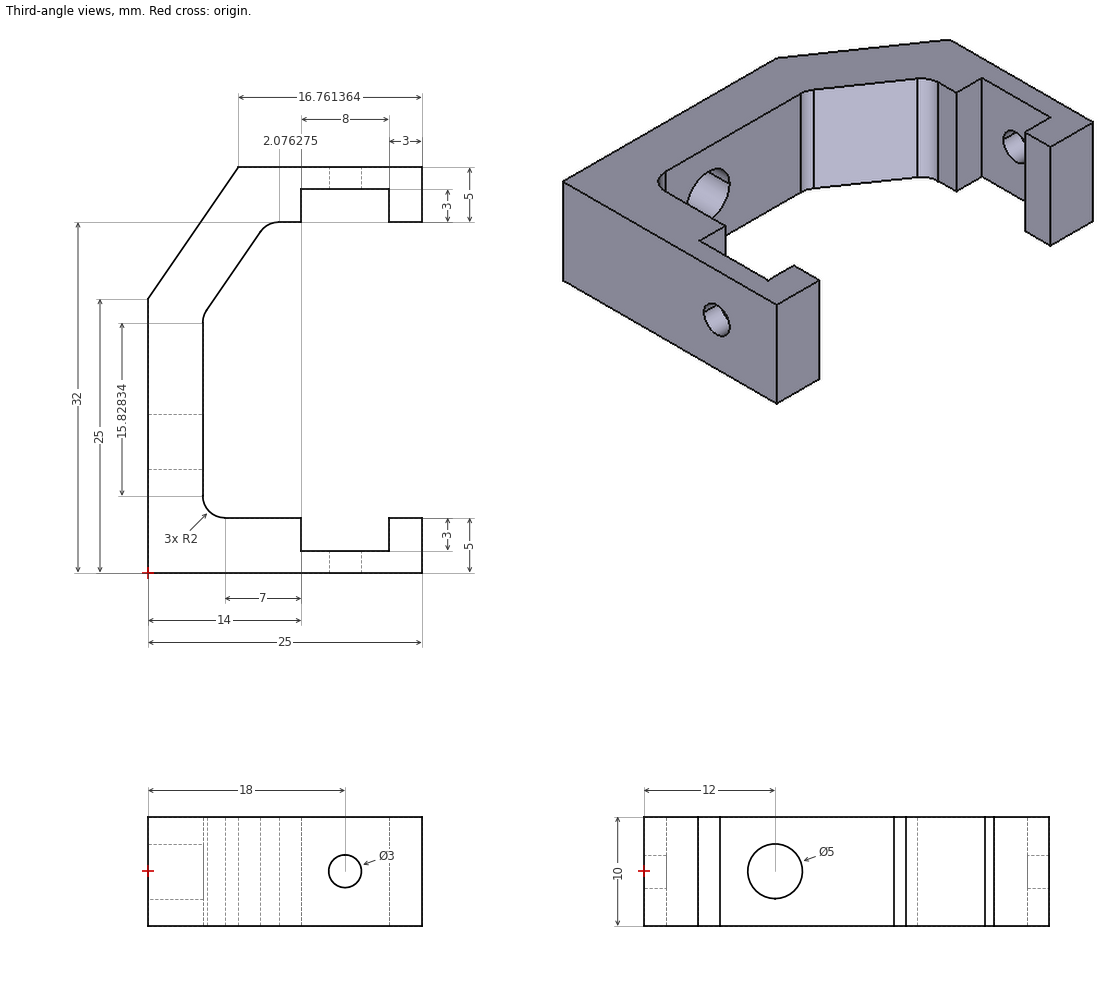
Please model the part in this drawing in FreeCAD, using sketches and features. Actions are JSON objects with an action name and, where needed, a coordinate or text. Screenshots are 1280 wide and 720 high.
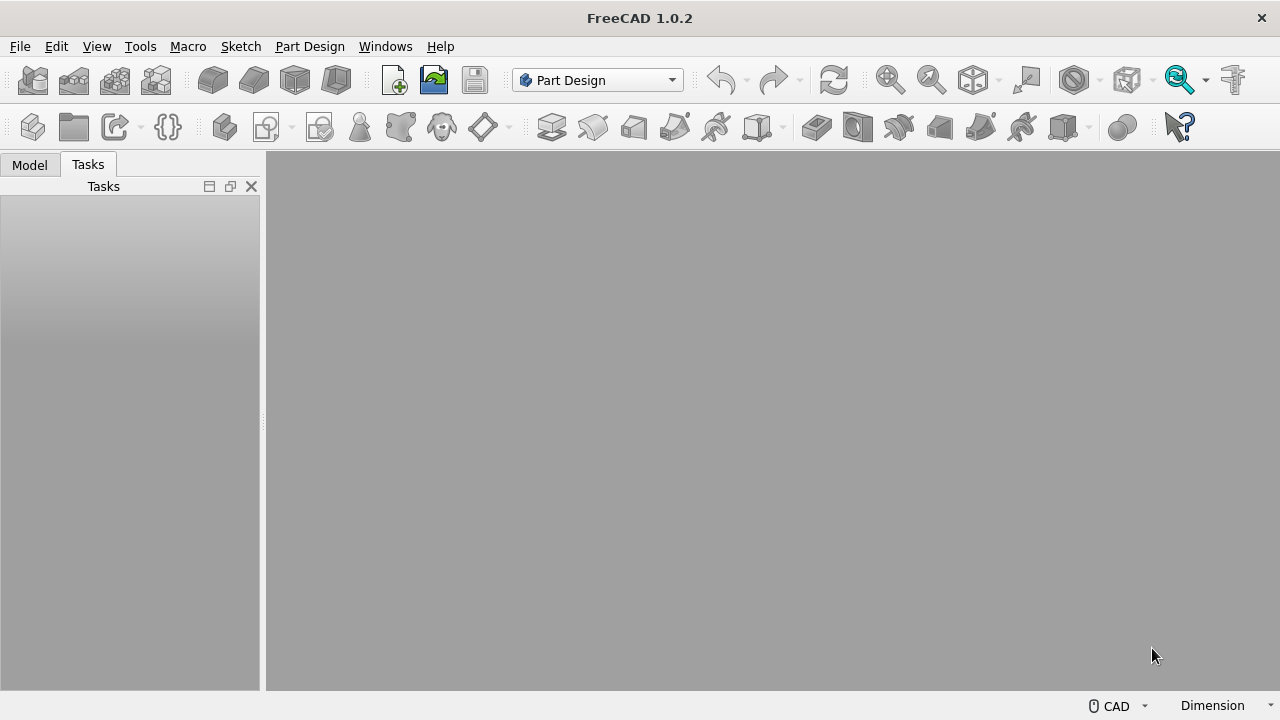
{"action": "left_click", "coordinate": [393, 80]}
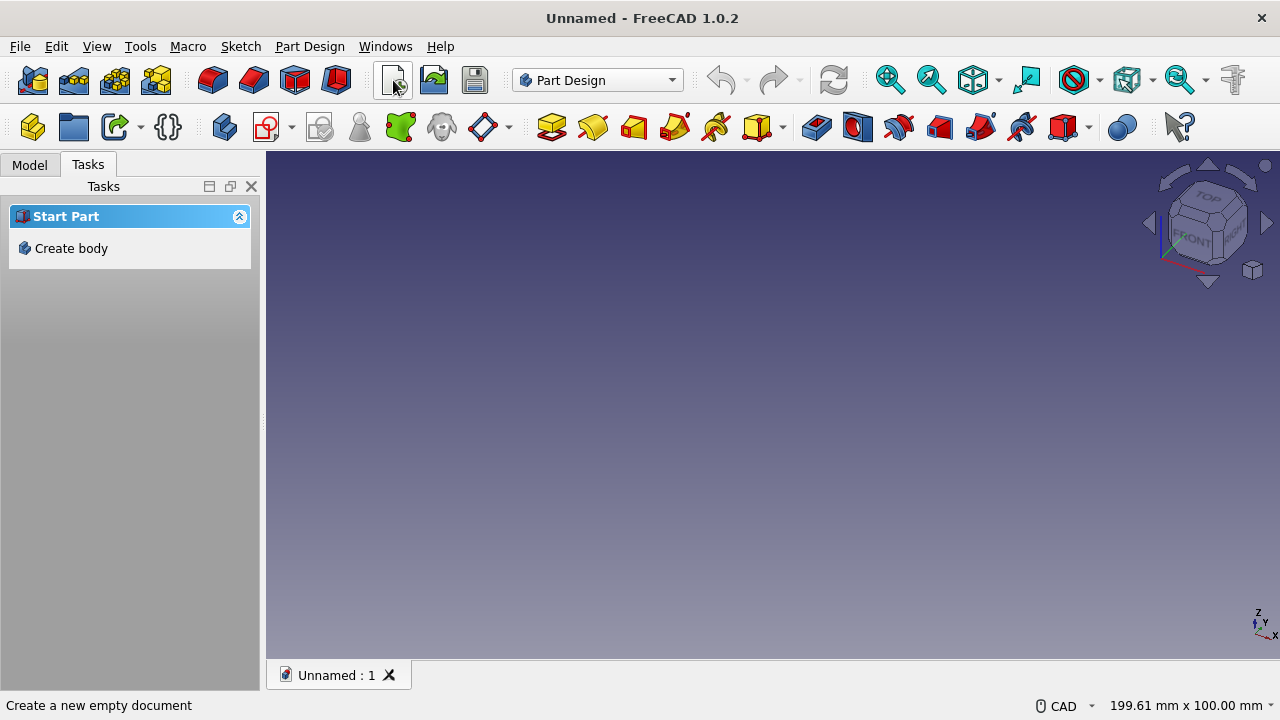
{"action": "left_click", "coordinate": [266, 128]}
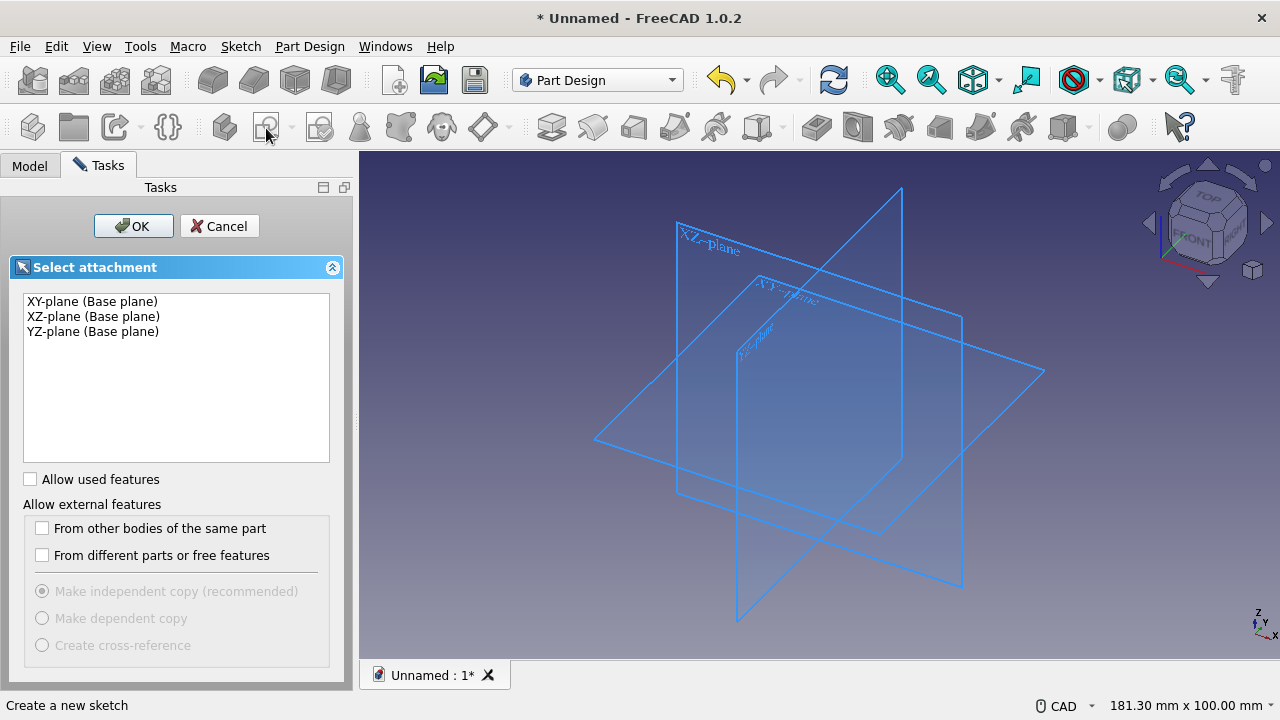
{"action": "left_click", "coordinate": [84, 302]}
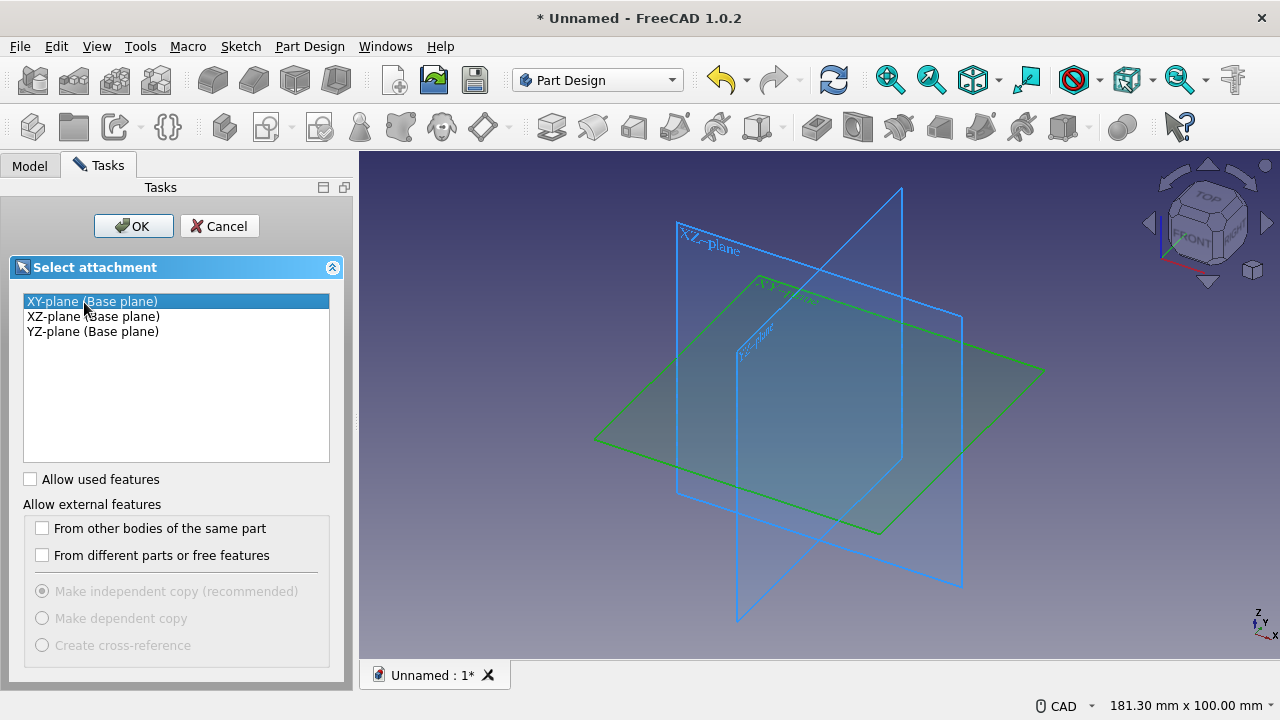
{"action": "left_click", "coordinate": [134, 226]}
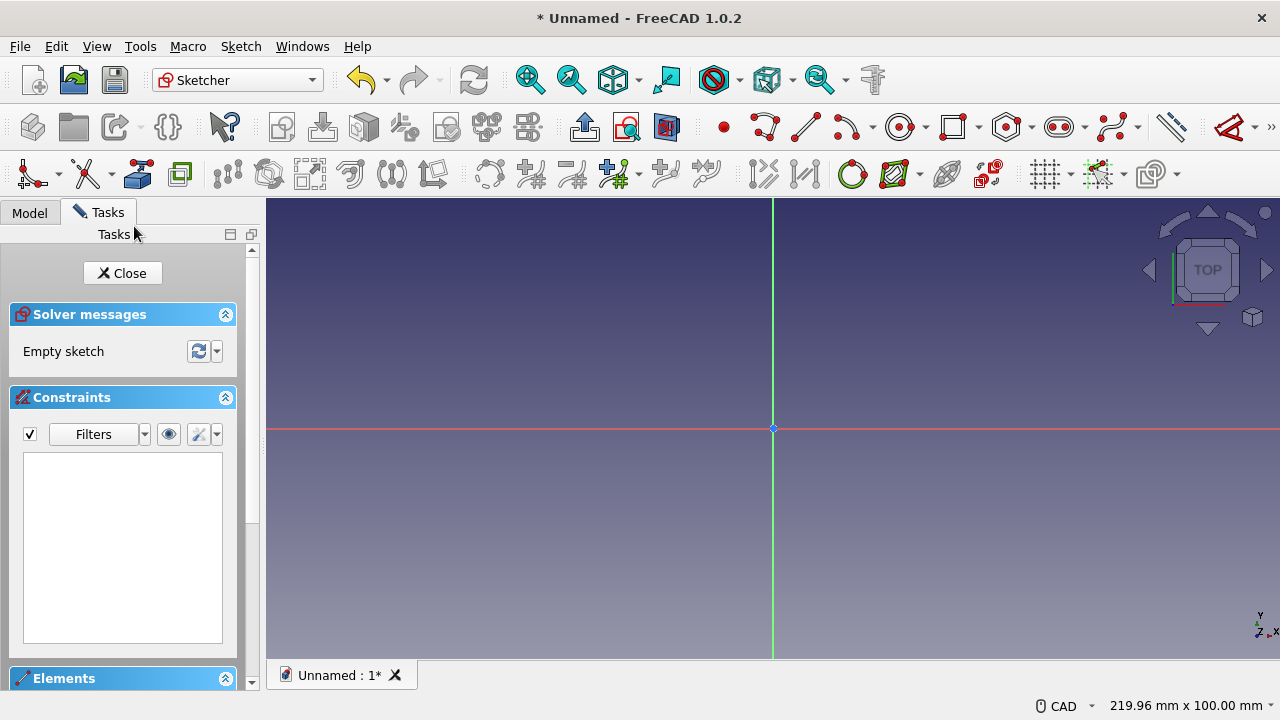
{"action": "scroll", "coordinate": [984, 239], "scroll_direction": "up", "scroll_amount": 3}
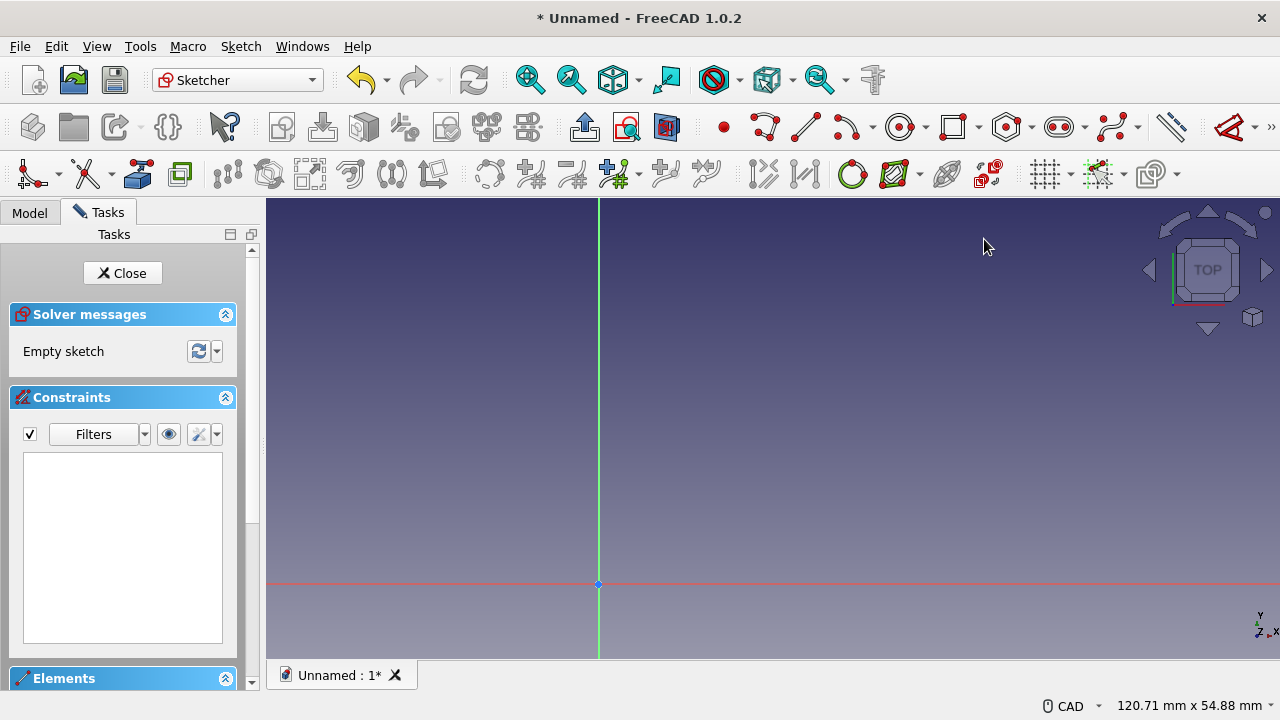
{"action": "left_click", "coordinate": [806, 128]}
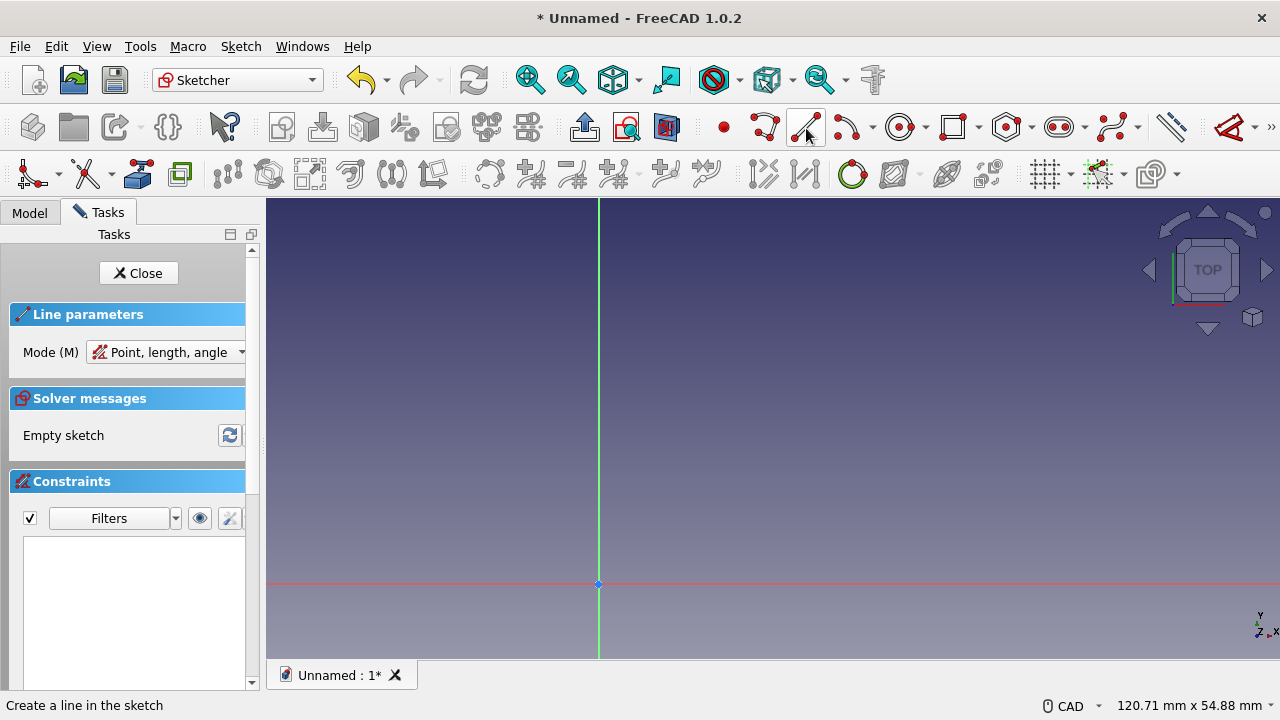
{"action": "left_click", "coordinate": [641, 525]}
{"action": "left_click", "coordinate": [641, 392]}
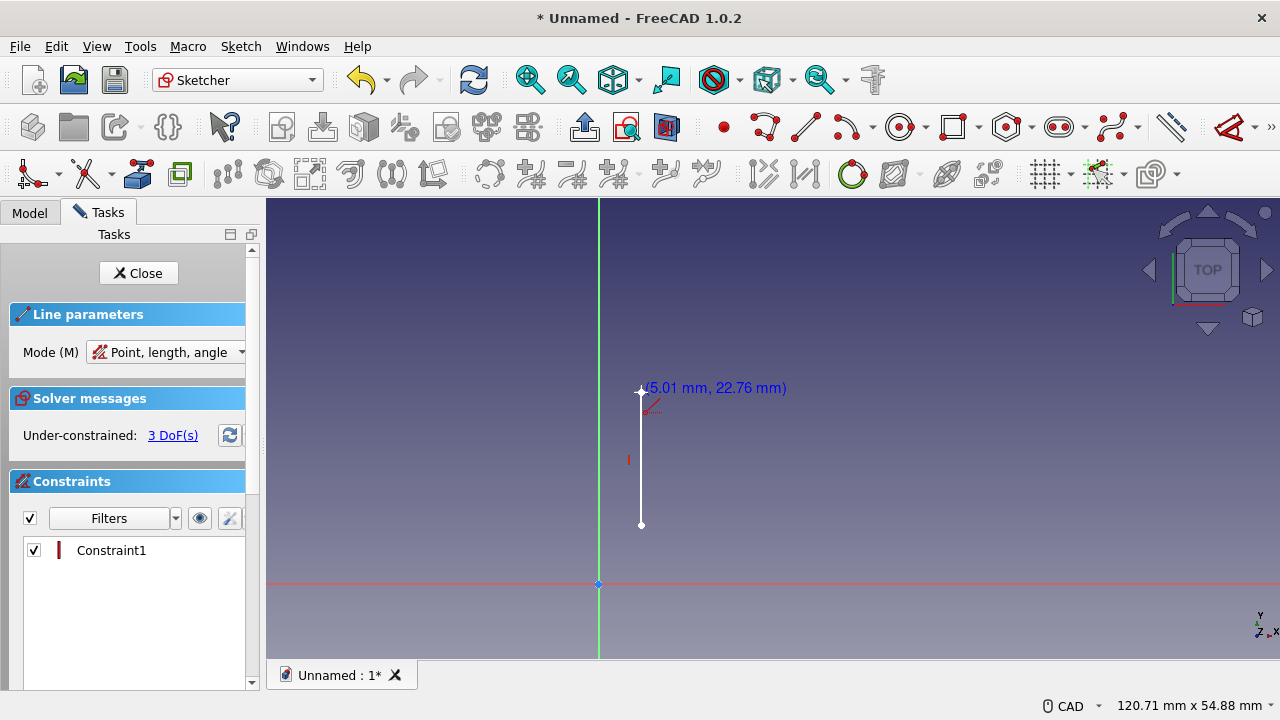
{"action": "scroll", "coordinate": [644, 383], "scroll_direction": "up", "scroll_amount": 3}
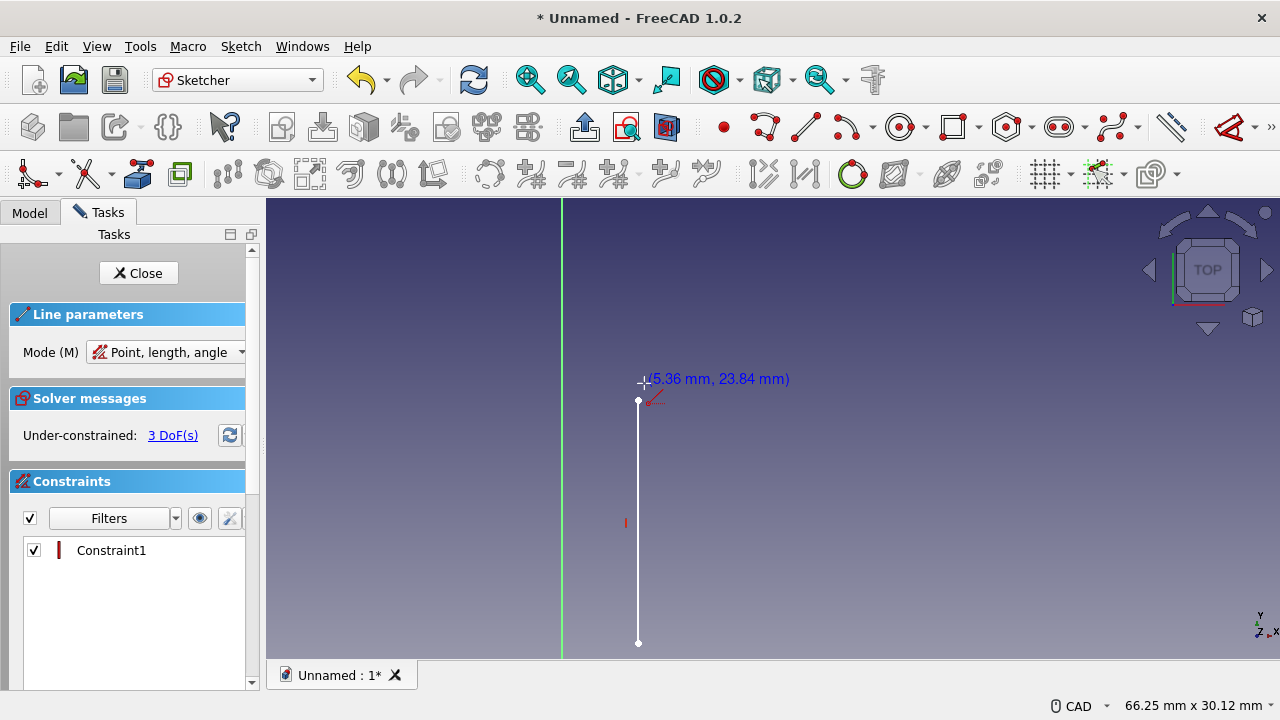
{"action": "left_click", "coordinate": [644, 383]}
{"action": "left_click", "coordinate": [719, 273]}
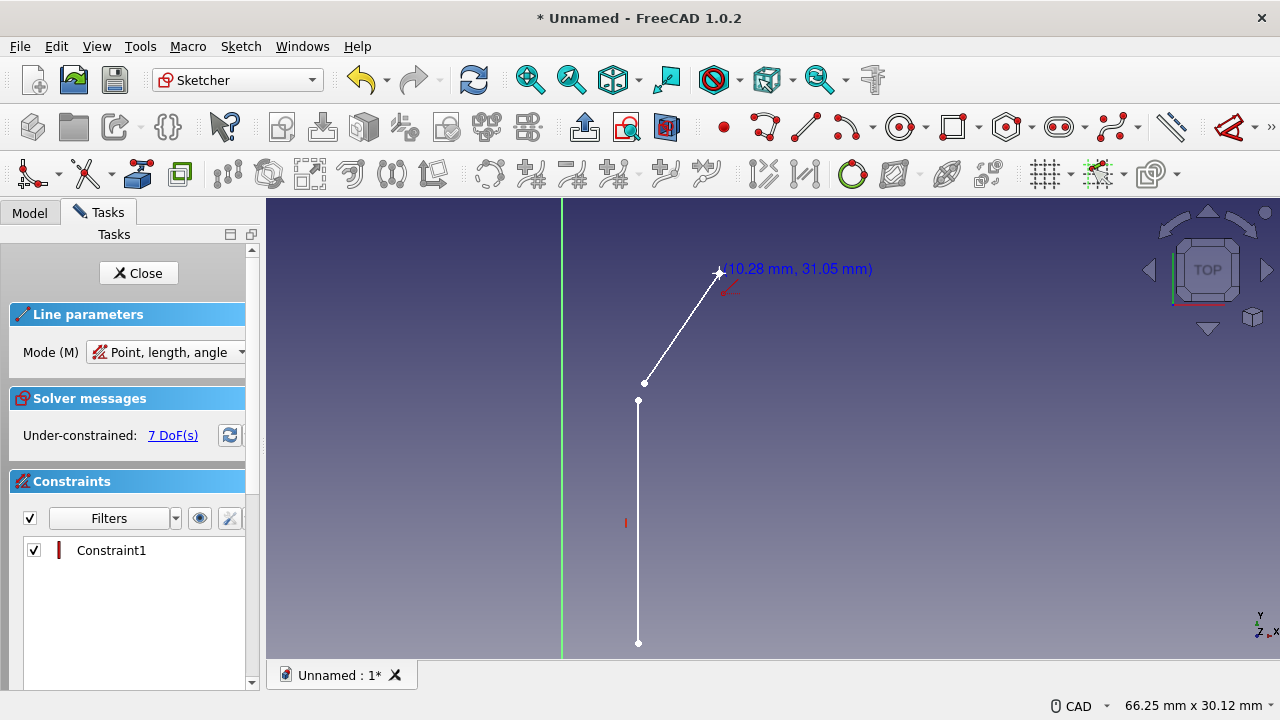
{"action": "left_click", "coordinate": [765, 128]}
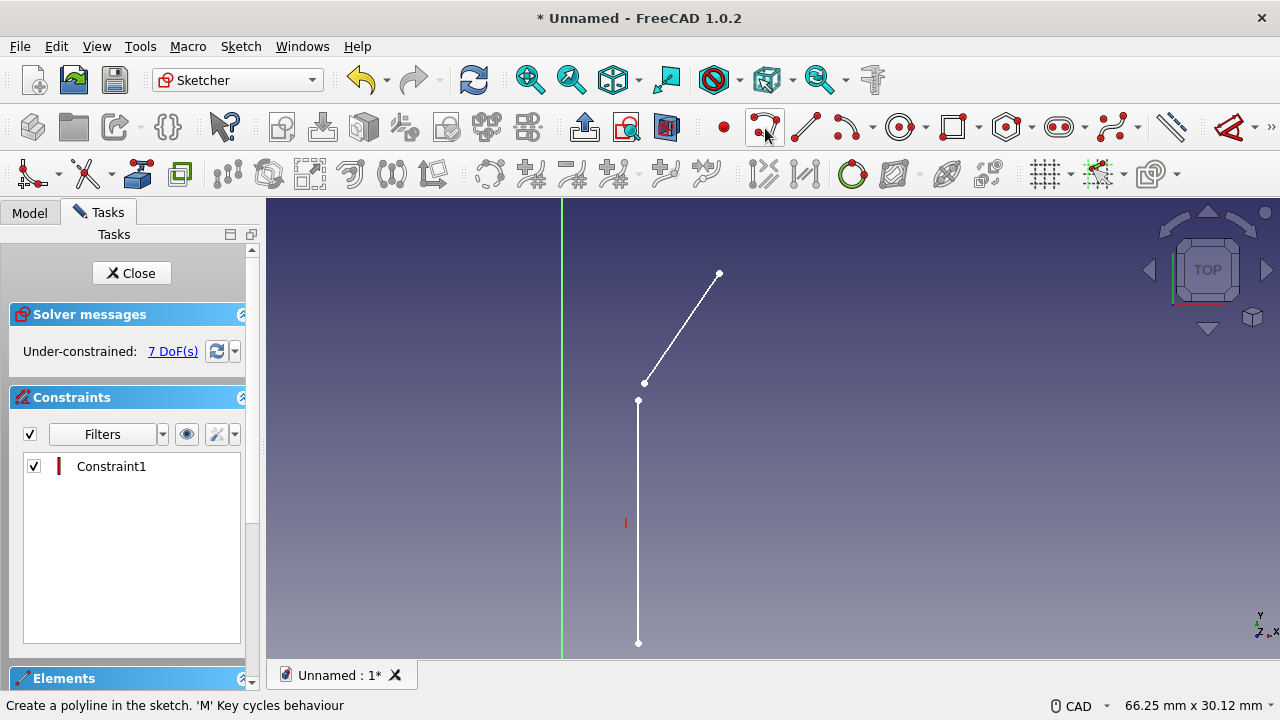
{"action": "left_click", "coordinate": [744, 260]}
{"action": "left_click", "coordinate": [776, 260]}